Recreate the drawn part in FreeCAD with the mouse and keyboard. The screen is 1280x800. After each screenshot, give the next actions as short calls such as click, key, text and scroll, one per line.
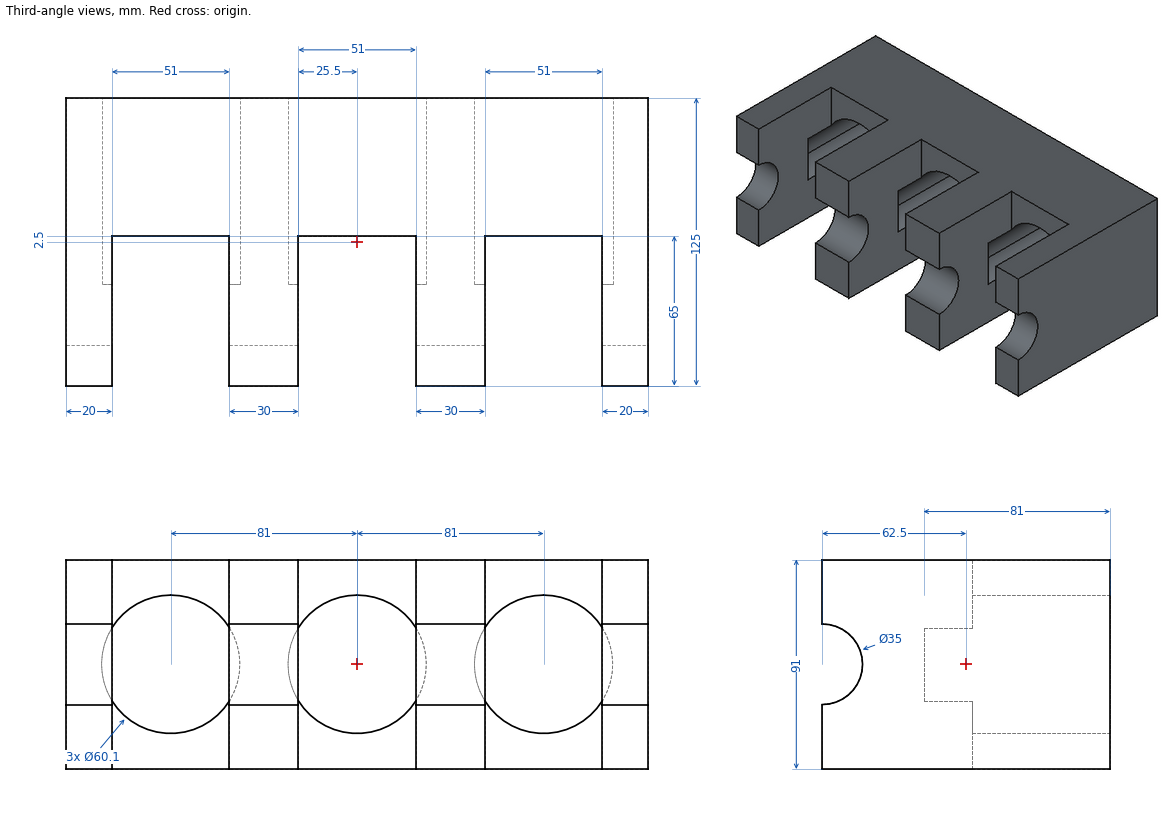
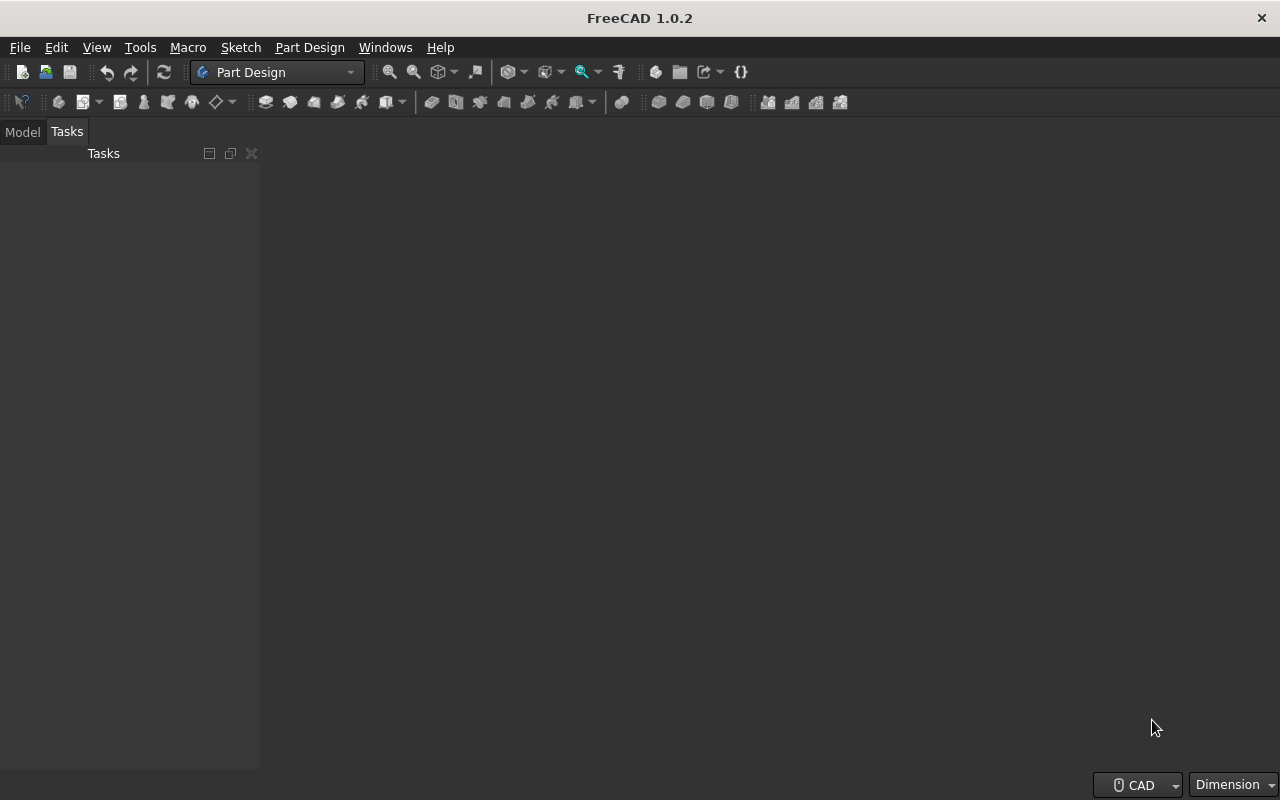
click(22, 72)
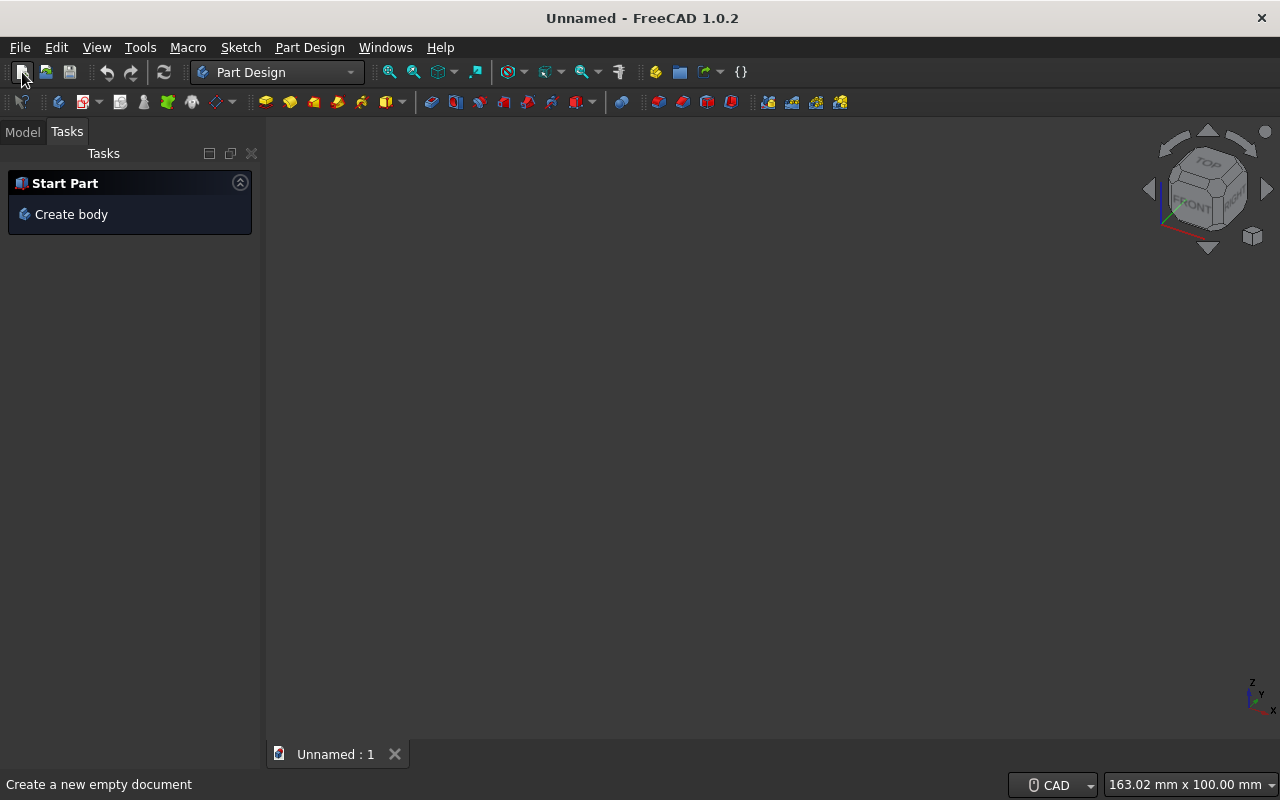
click(84, 102)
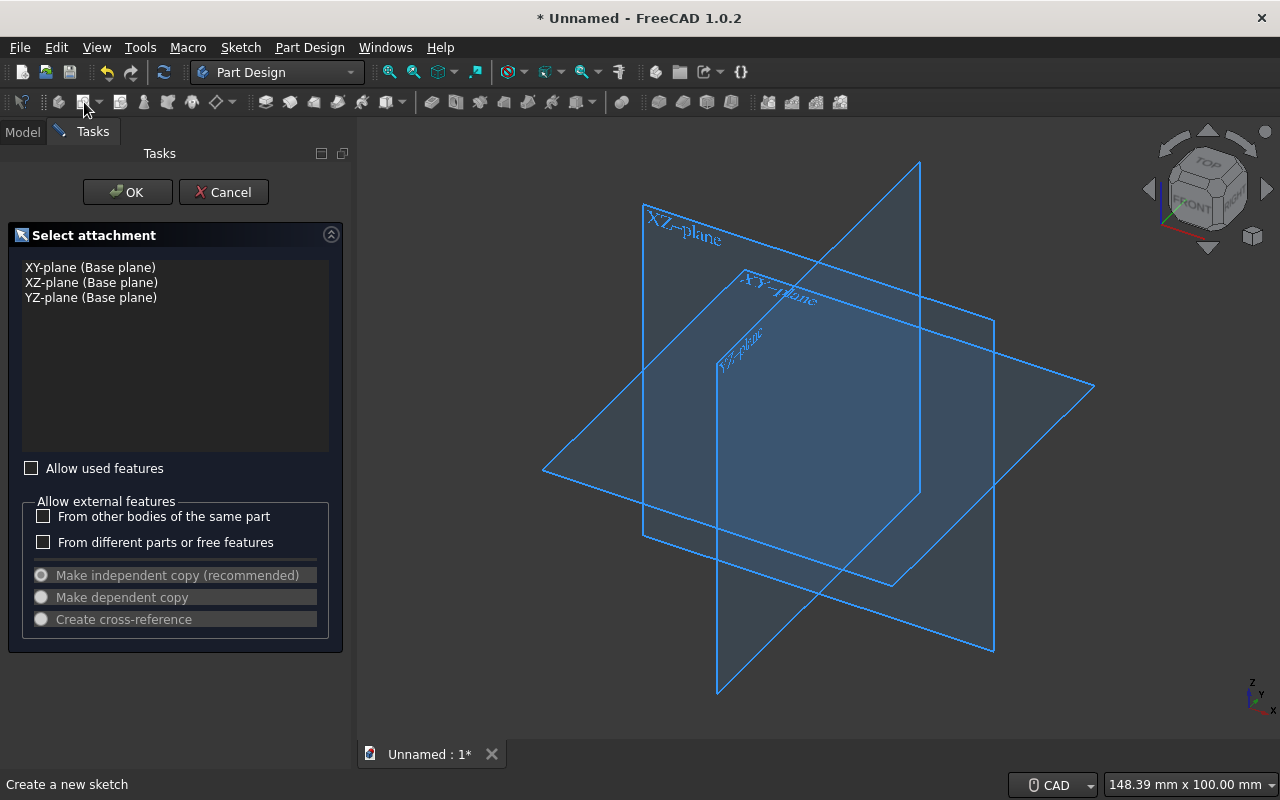
click(82, 268)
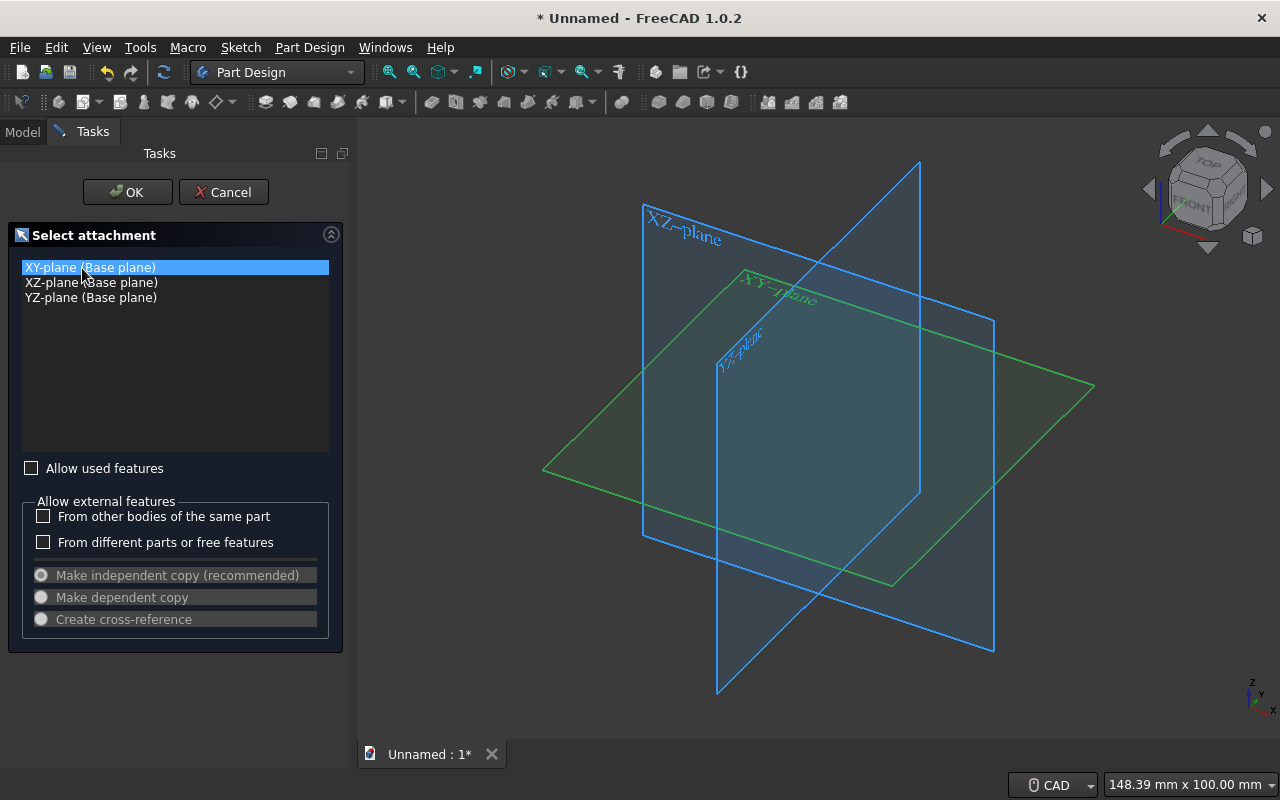
click(128, 192)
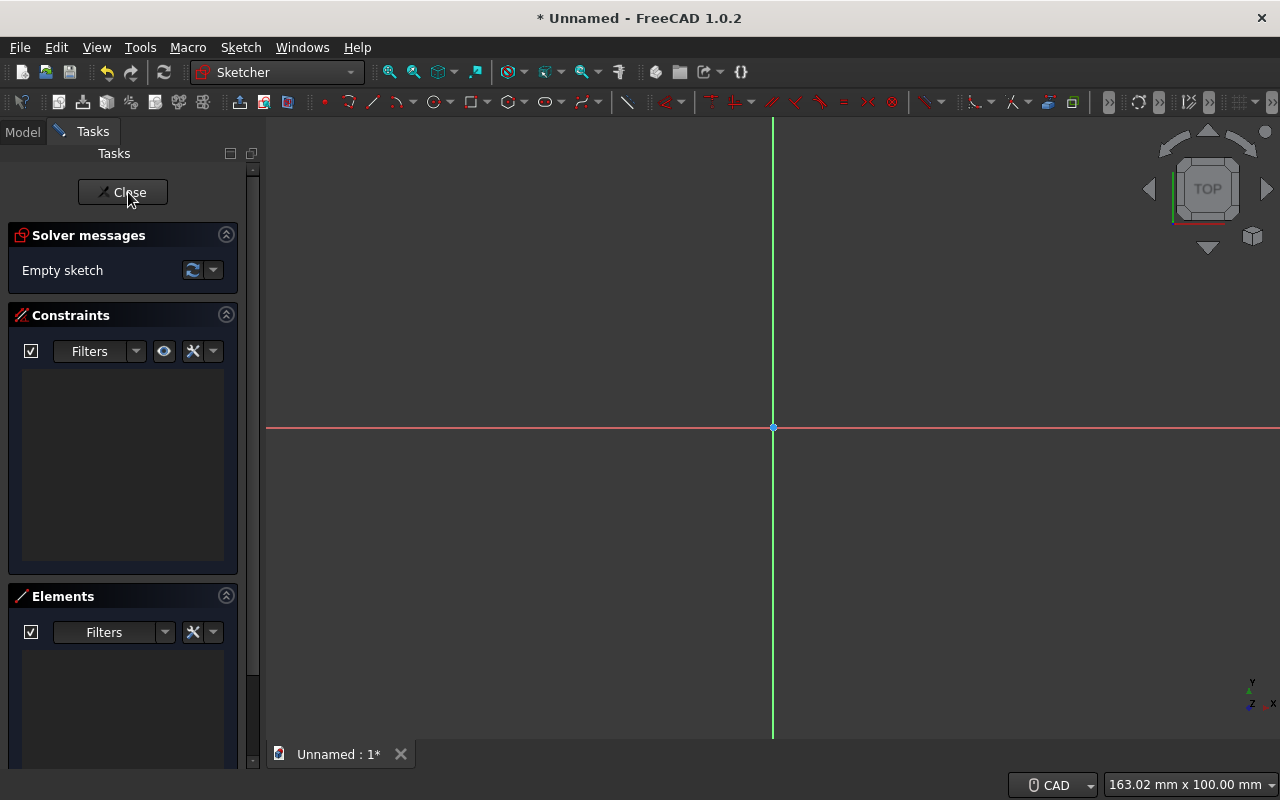
scroll(665, 428, down, 5)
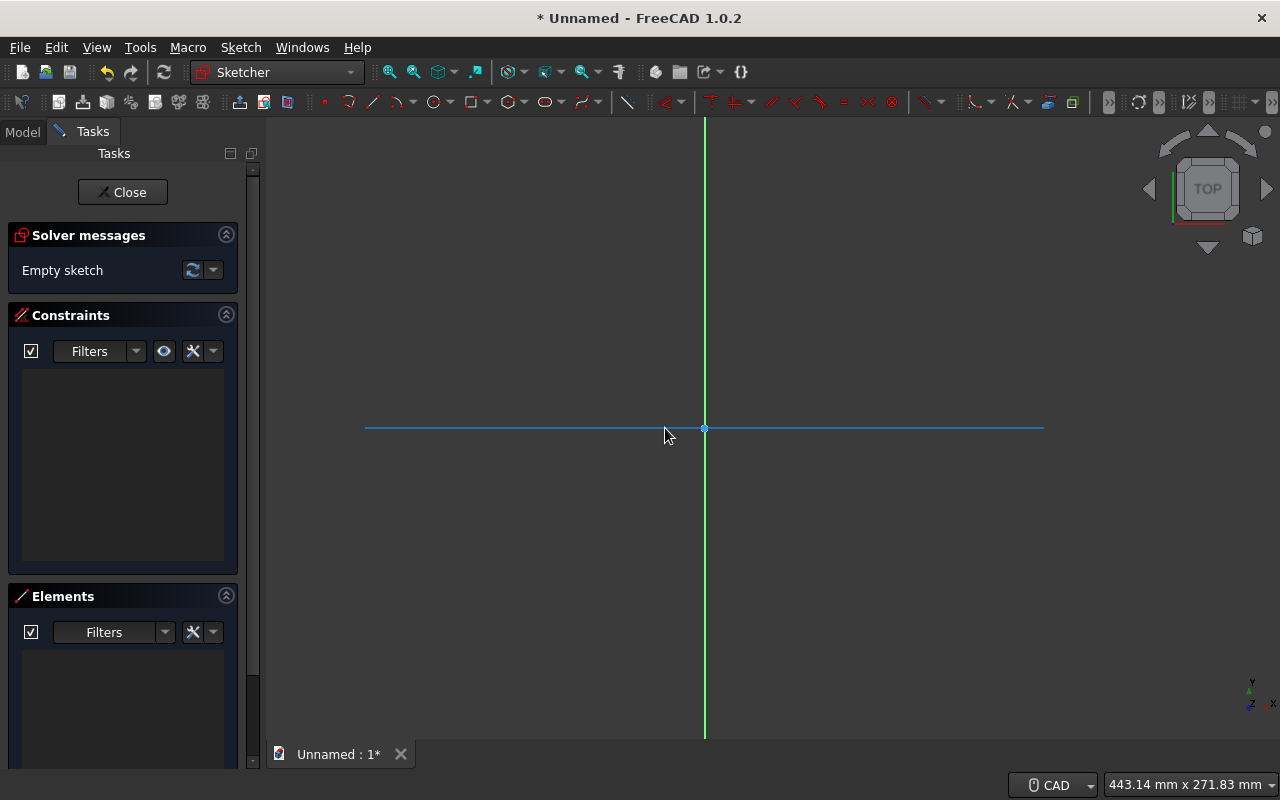
click(350, 102)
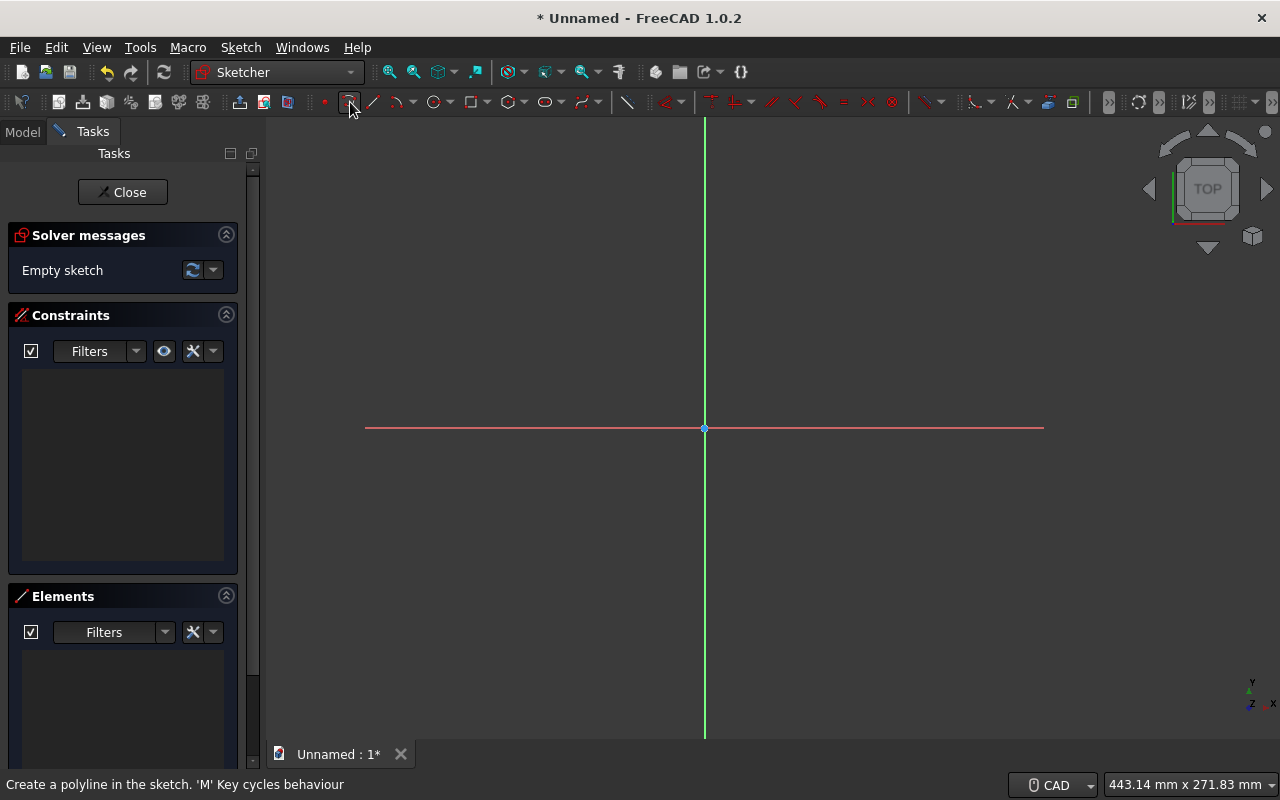
scroll(647, 423, up, 6)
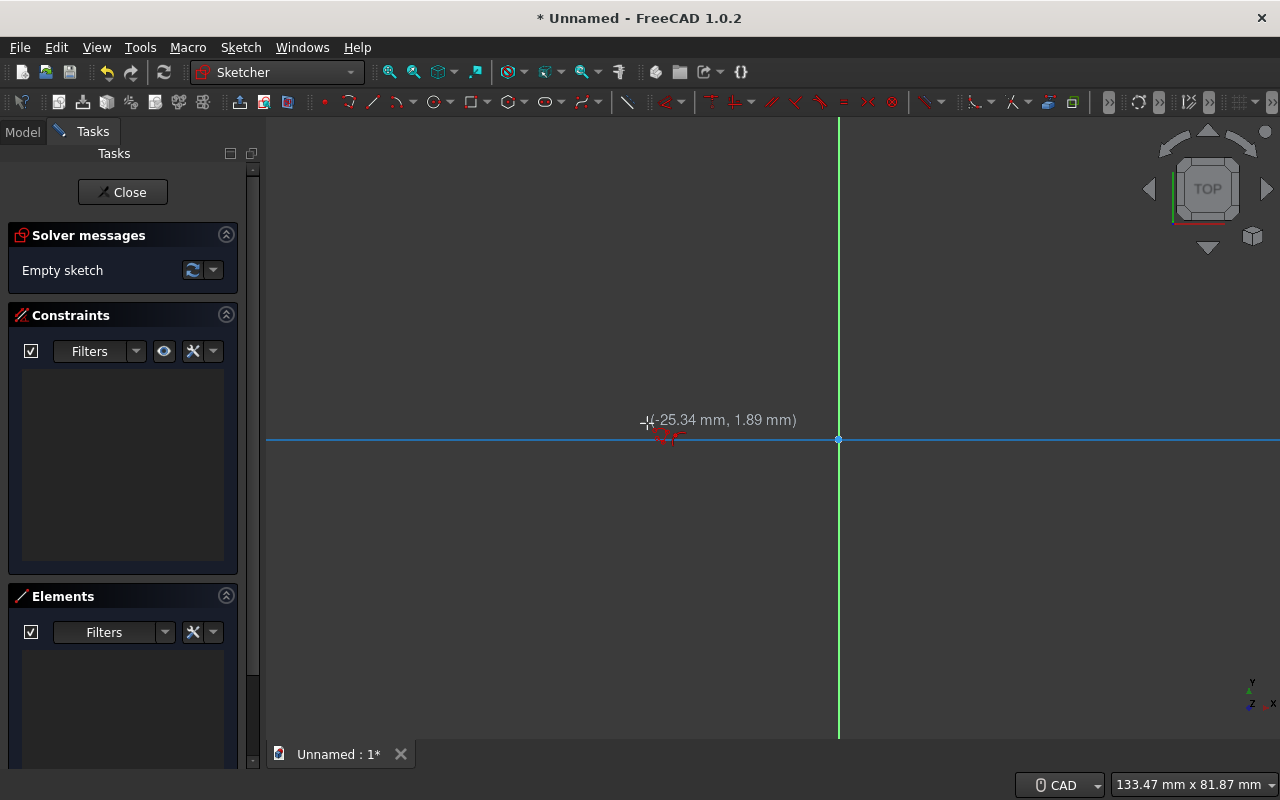
click(645, 421)
click(1032, 421)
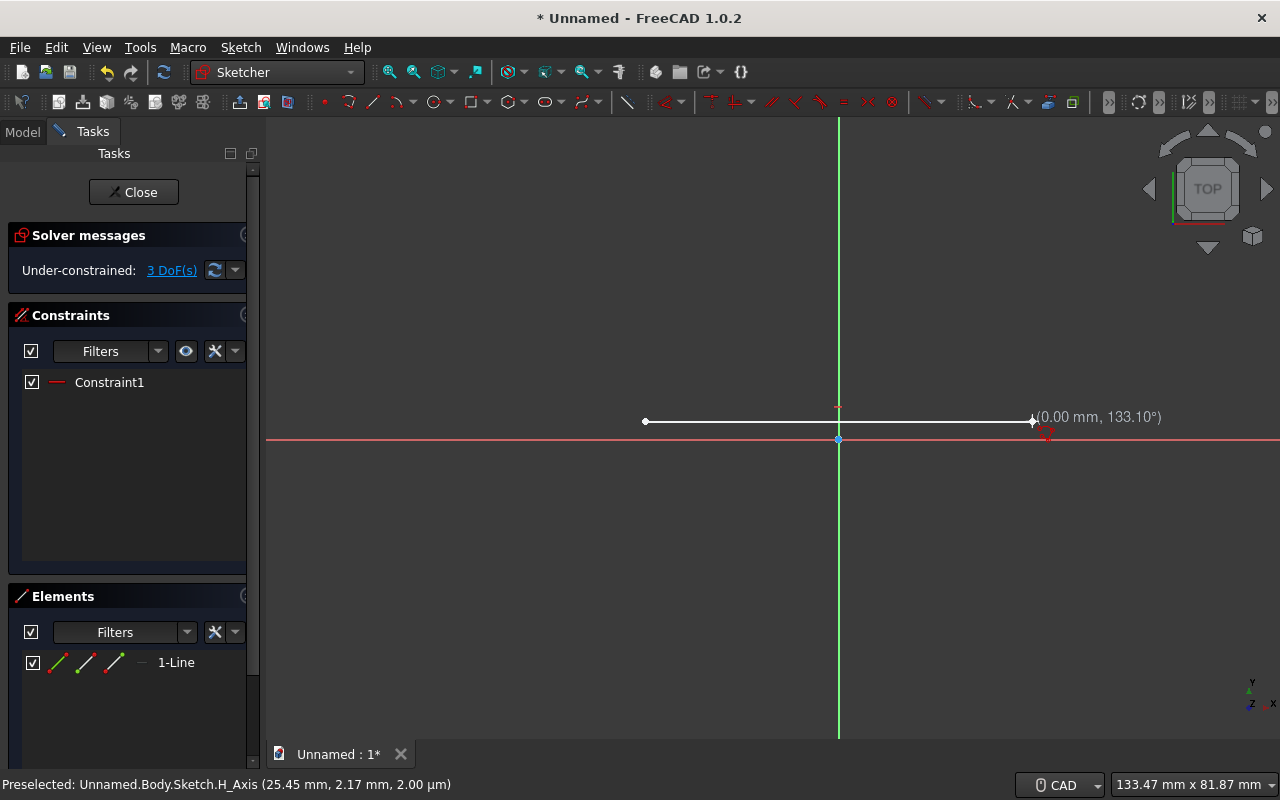
scroll(647, 423, down, 6)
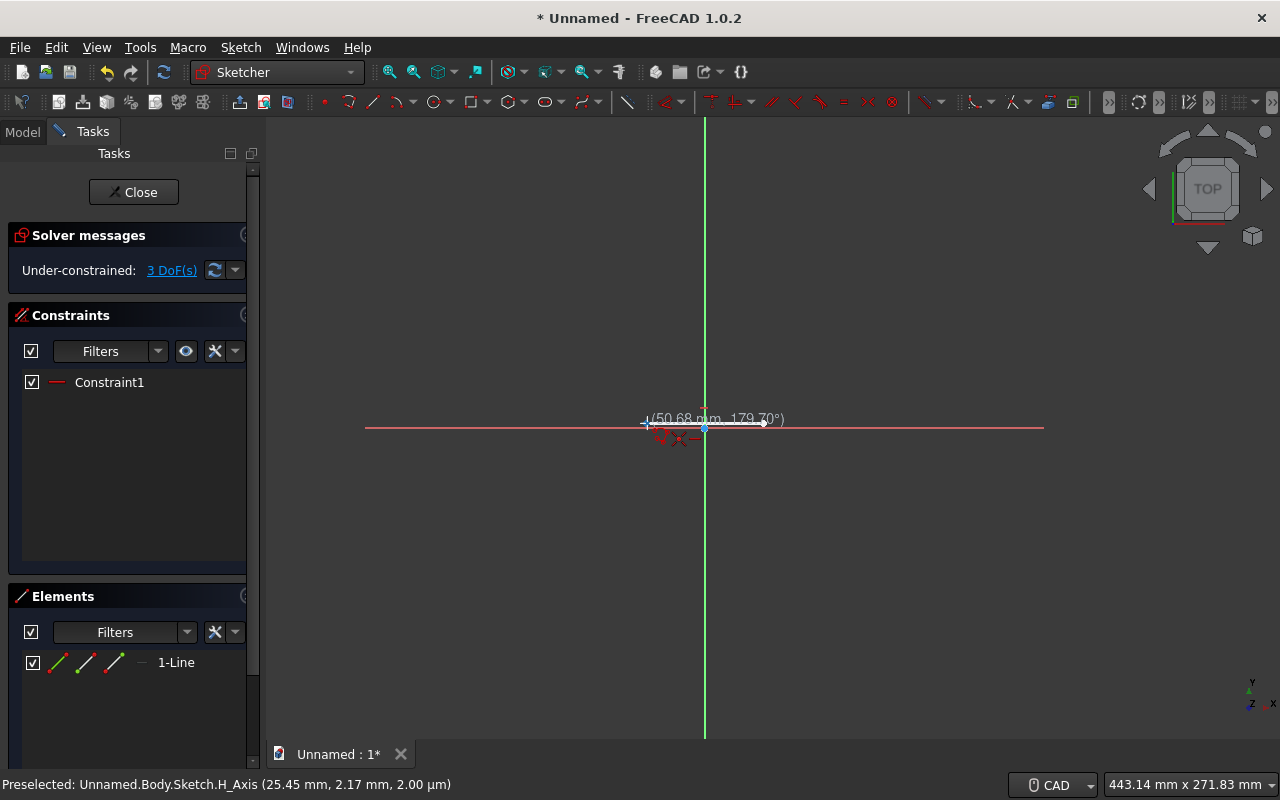
click(763, 571)
click(832, 571)